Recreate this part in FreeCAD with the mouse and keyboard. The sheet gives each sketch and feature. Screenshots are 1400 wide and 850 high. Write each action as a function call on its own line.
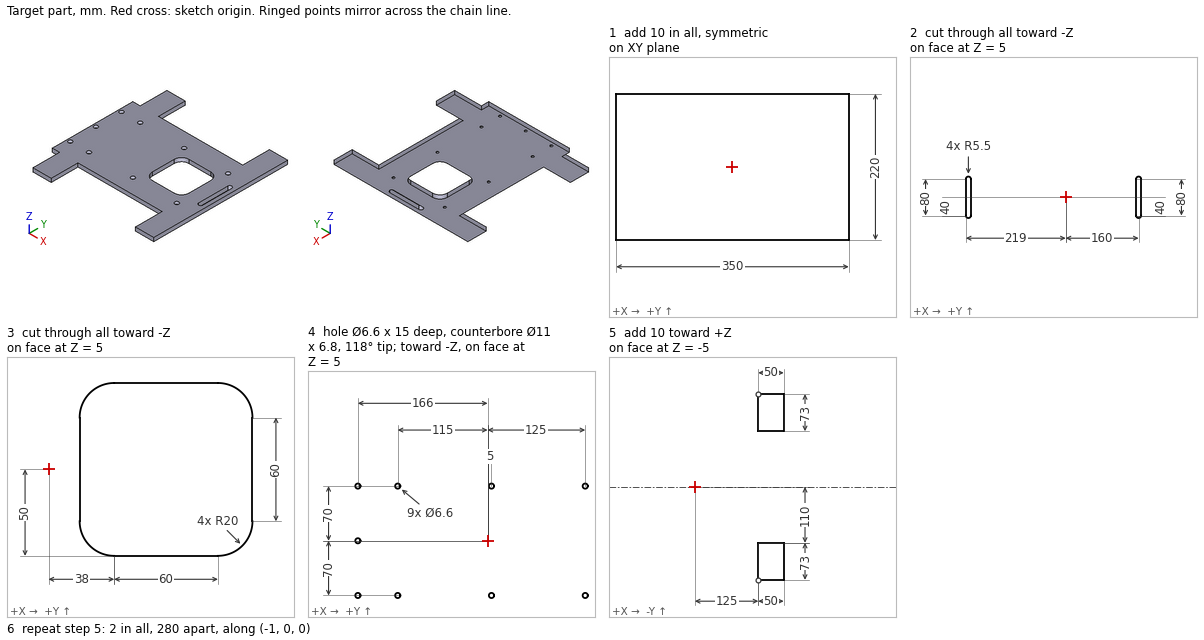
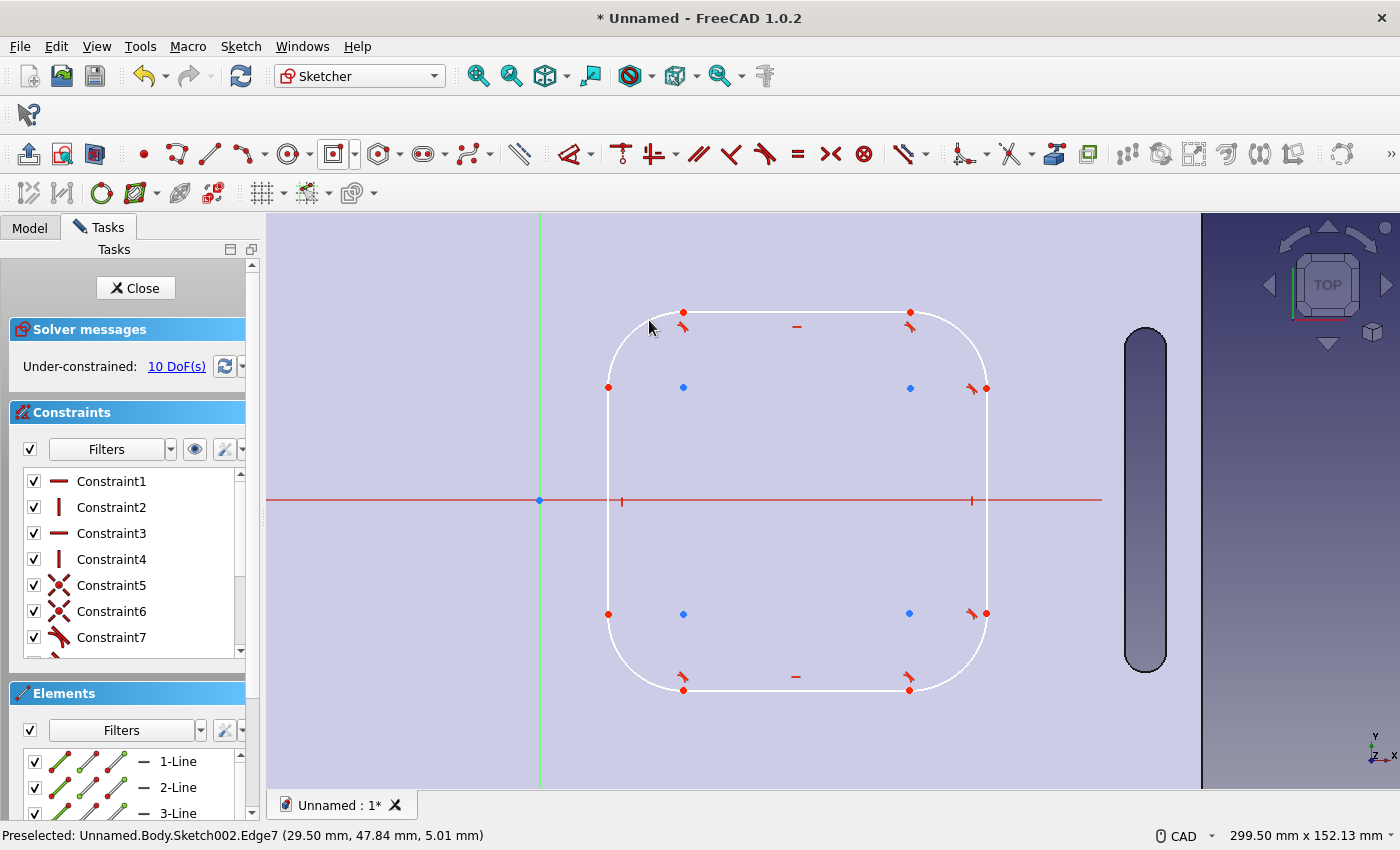
click(608, 456)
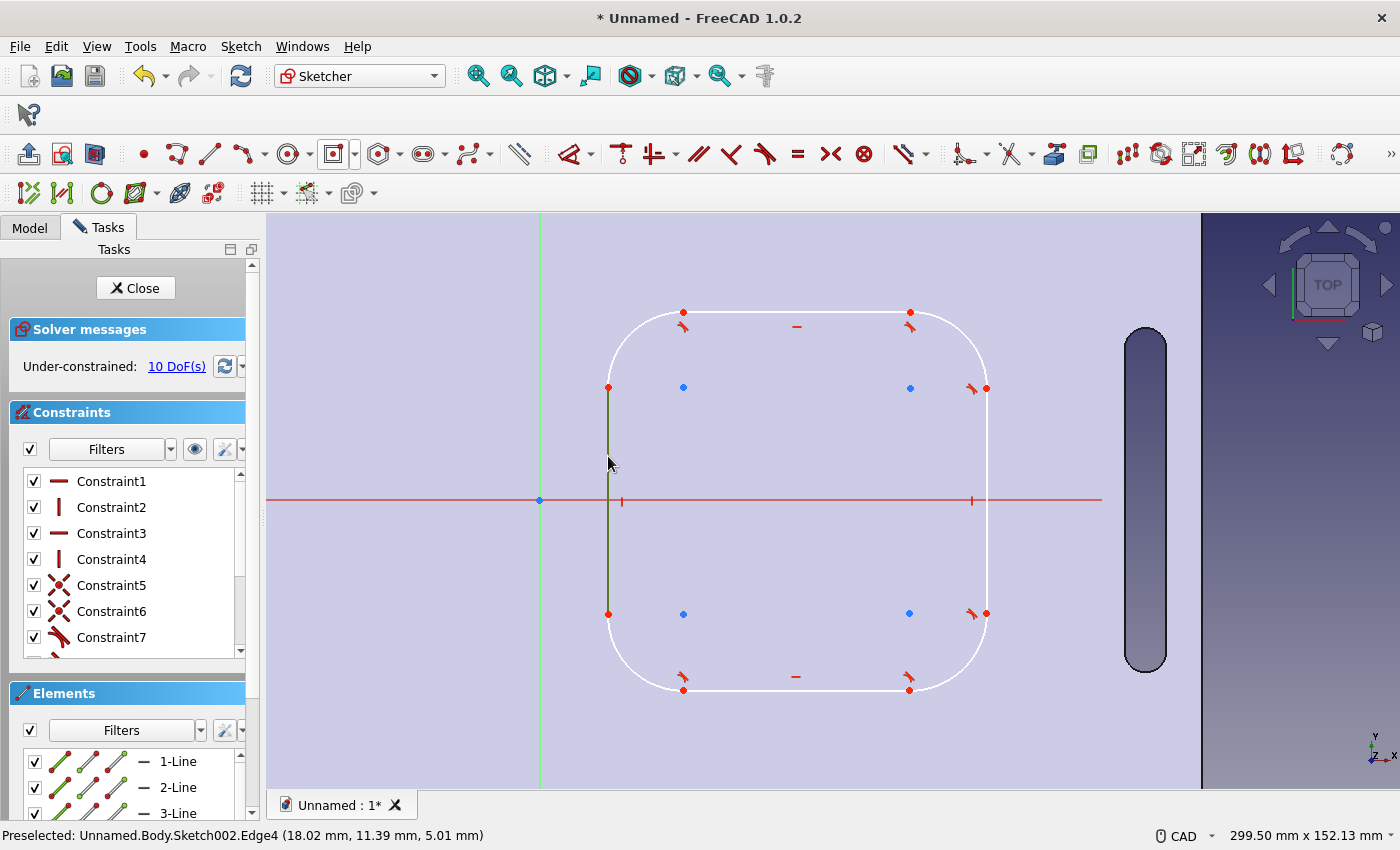
click(650, 320)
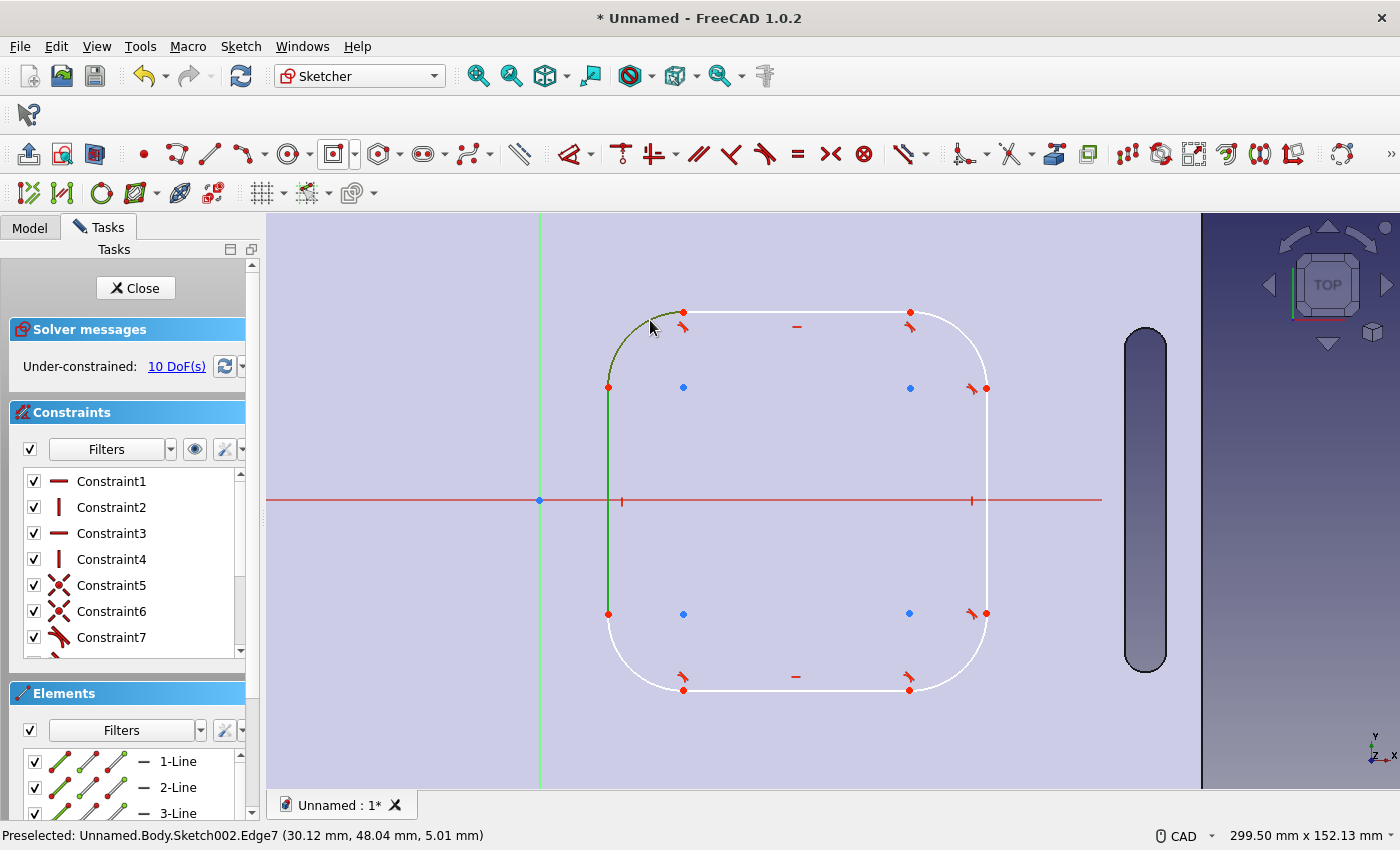
click(765, 154)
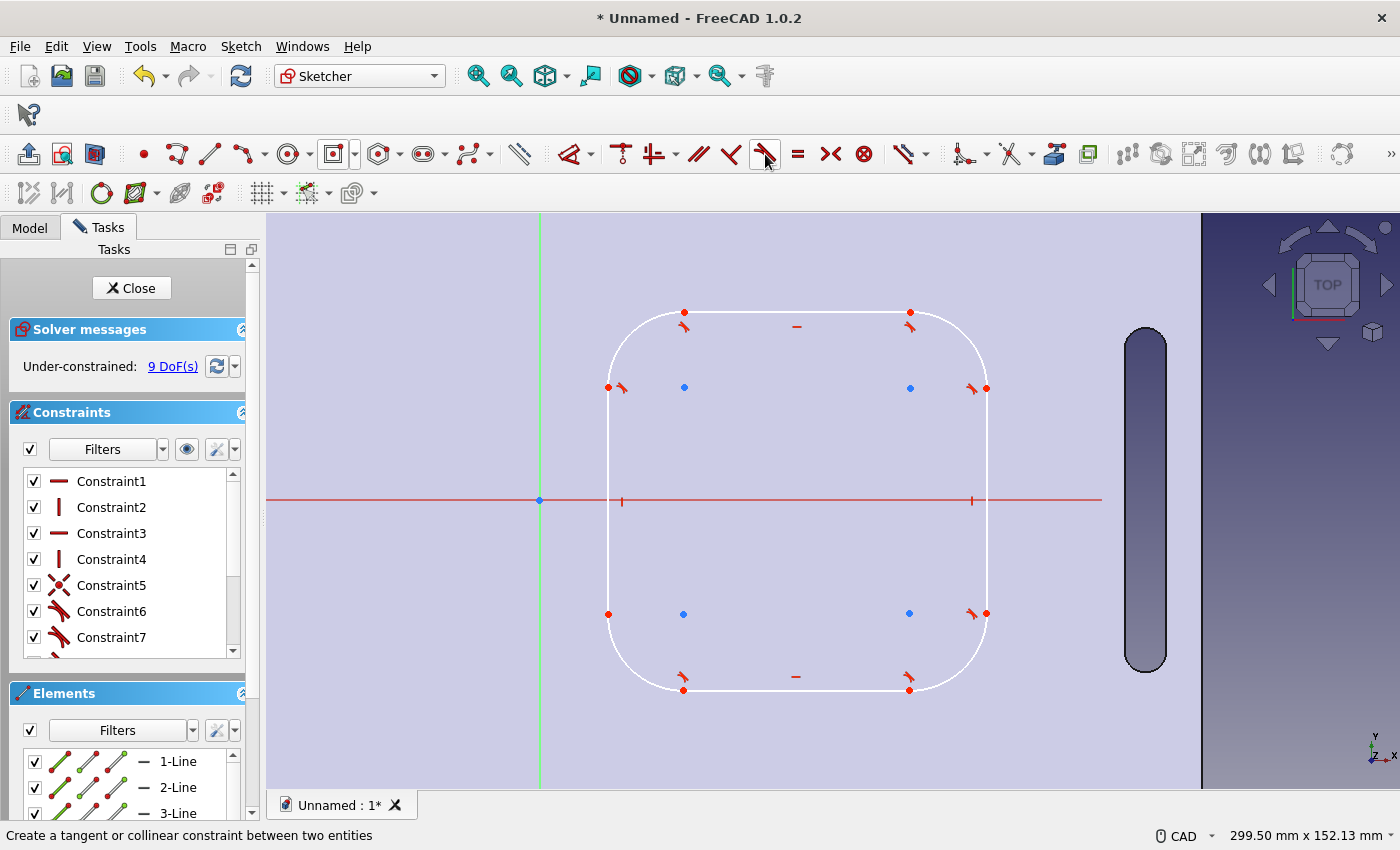
click(608, 456)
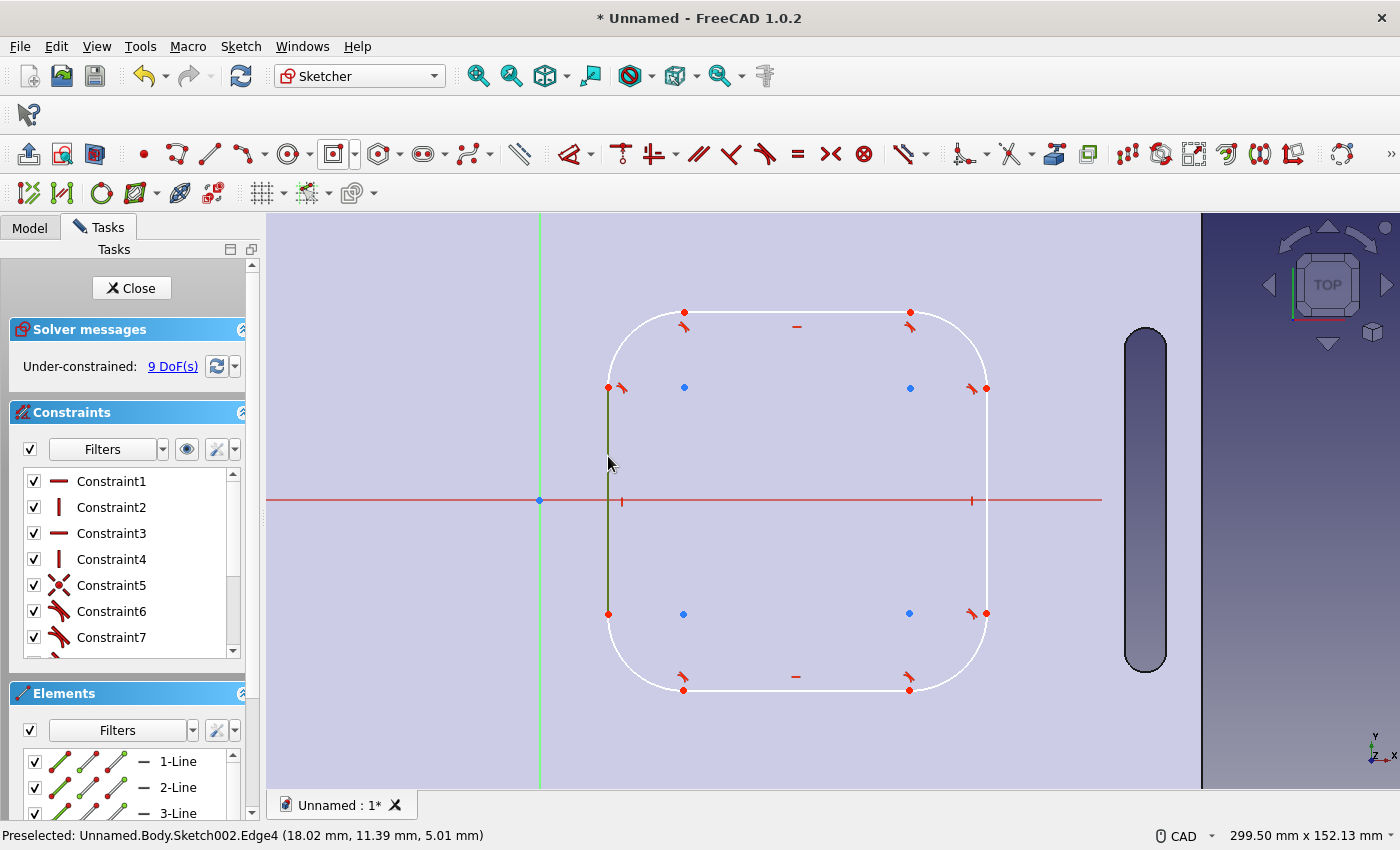
click(616, 649)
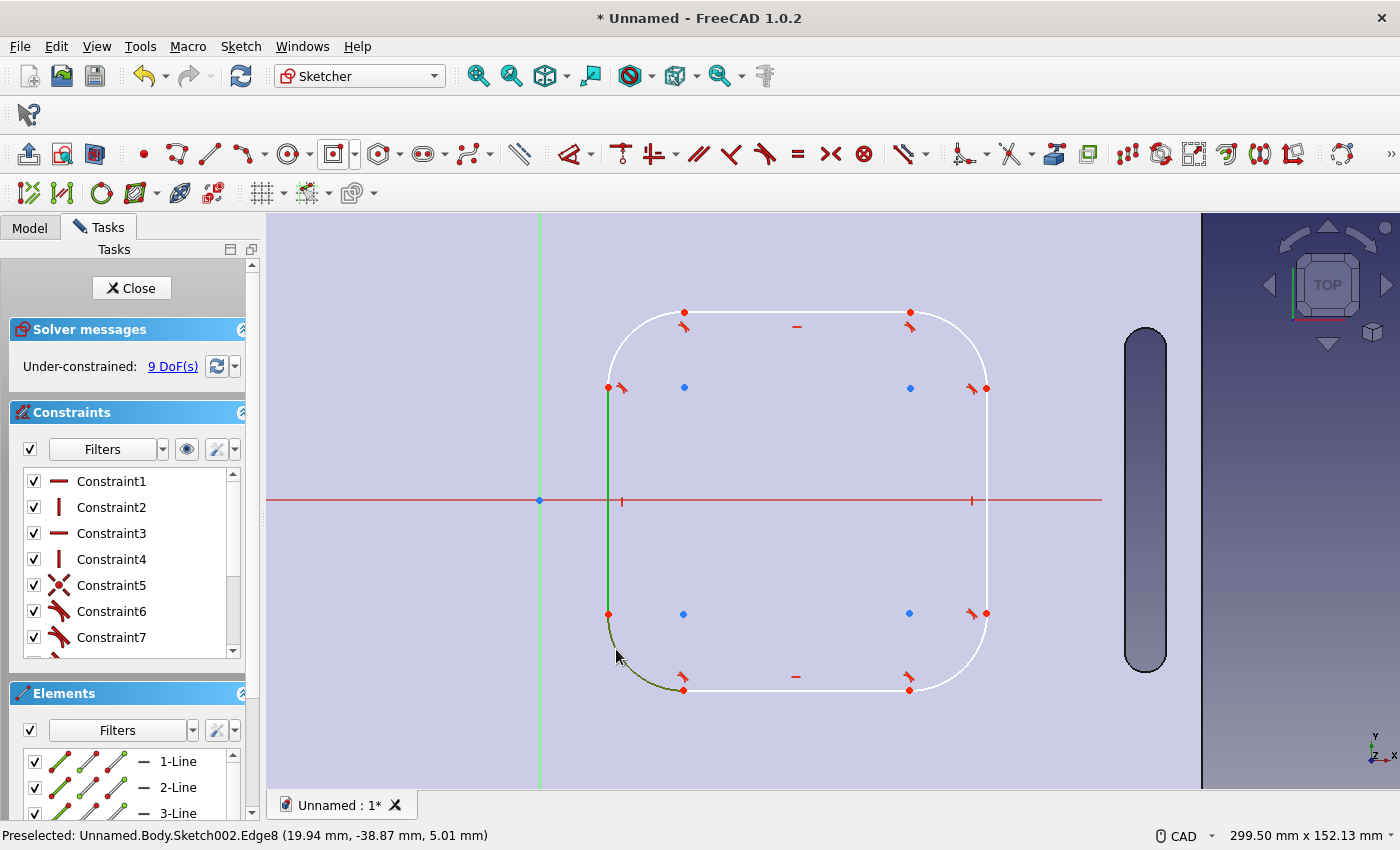
click(765, 154)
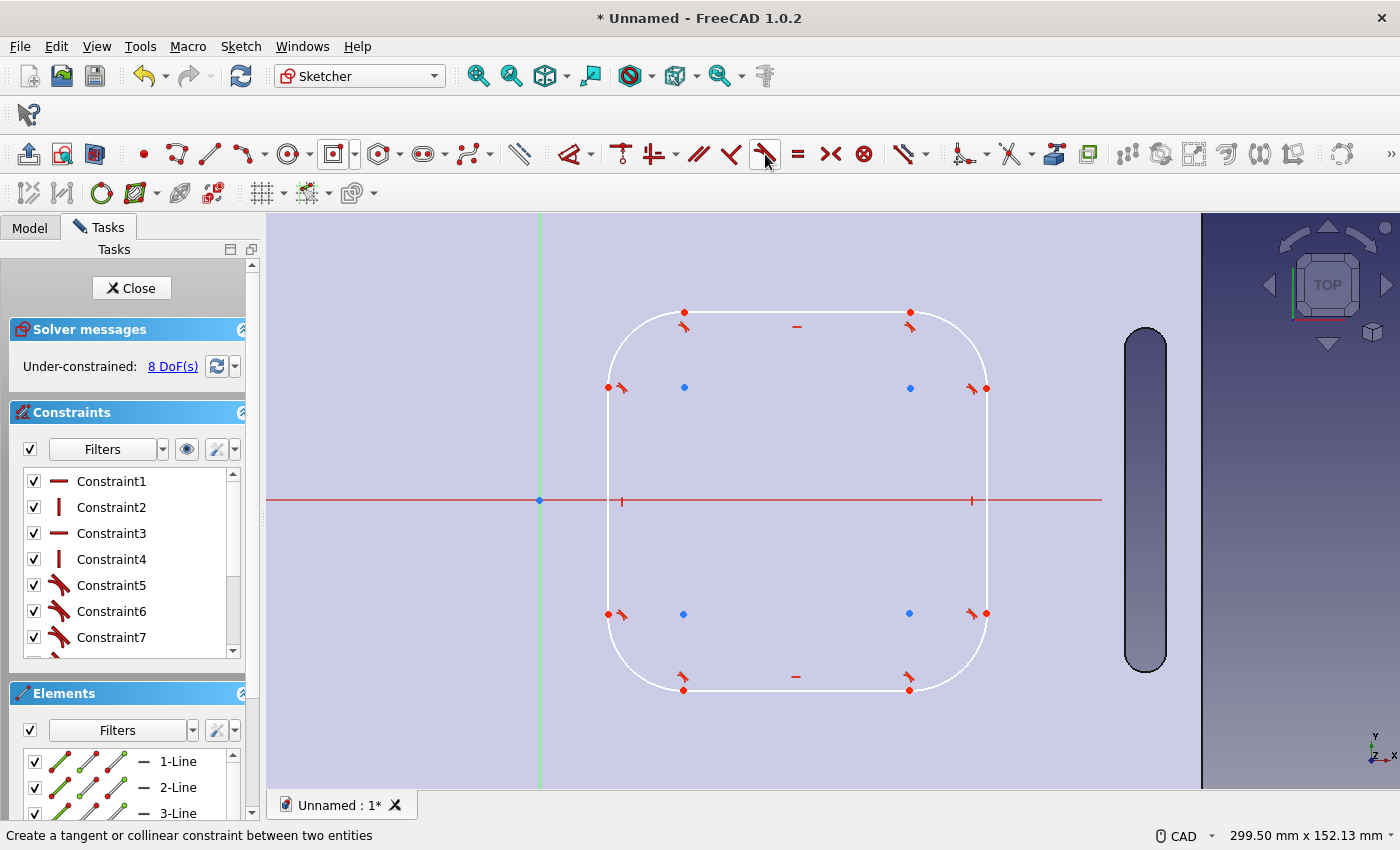
click(945, 682)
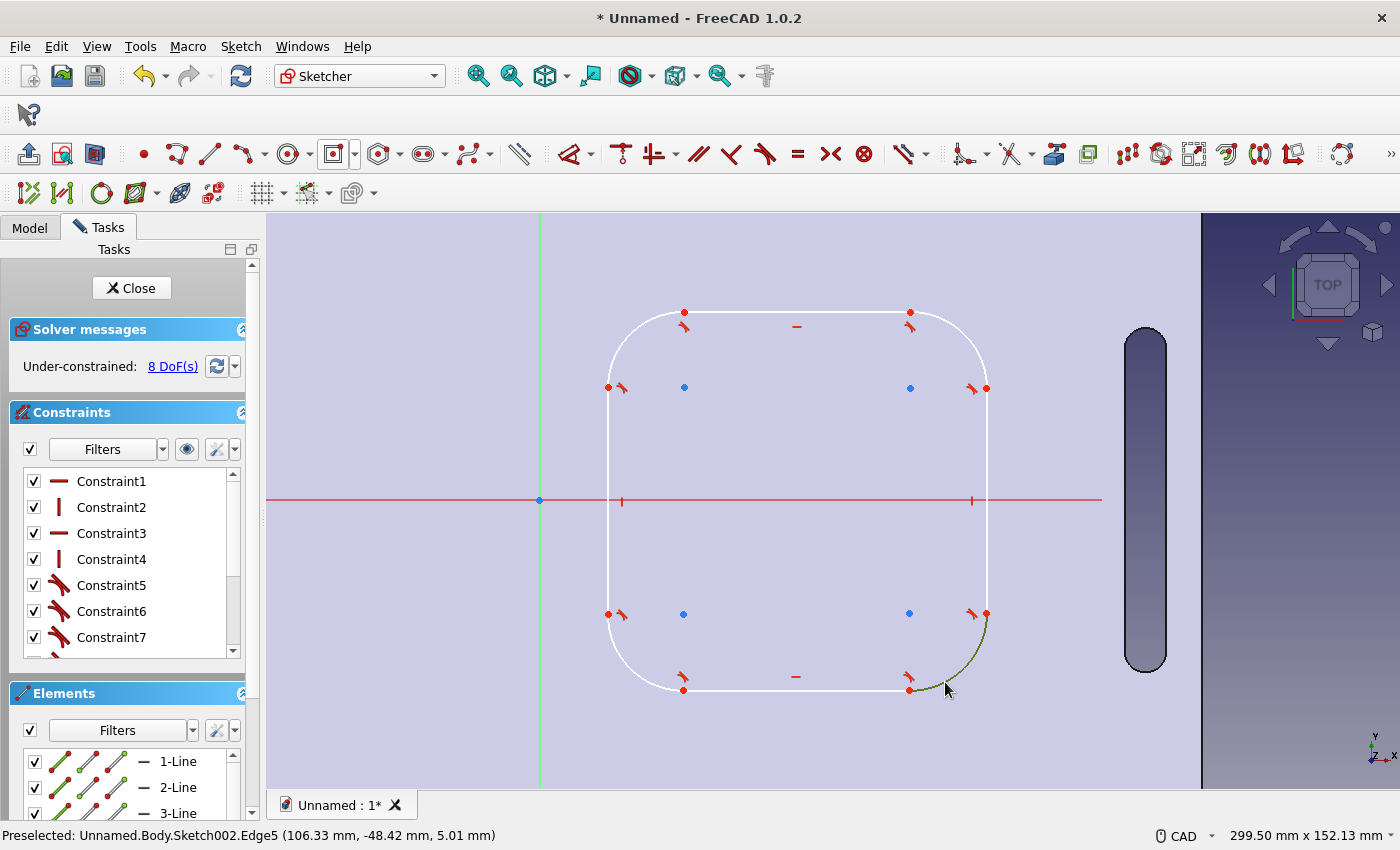
click(979, 354)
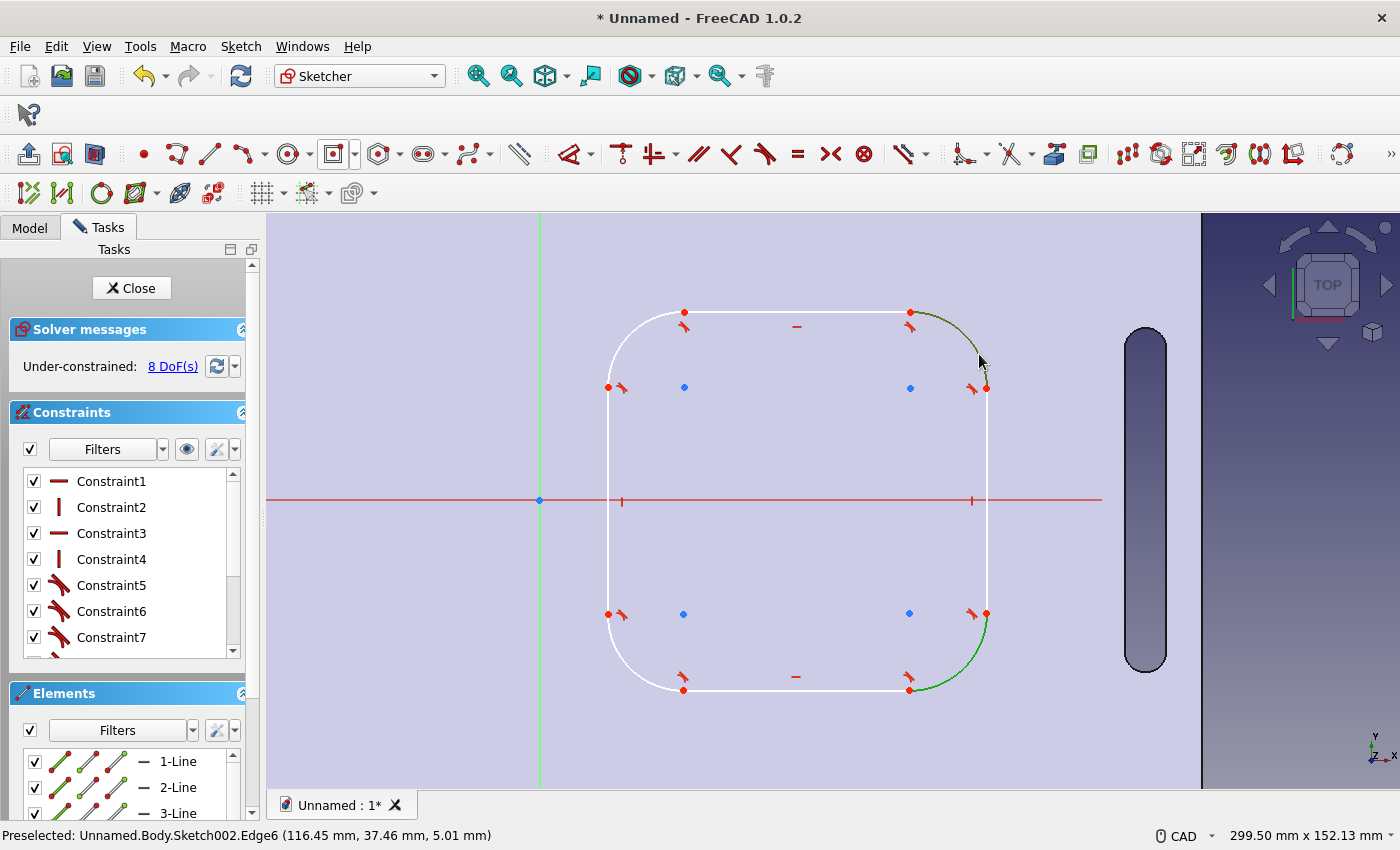
click(650, 320)